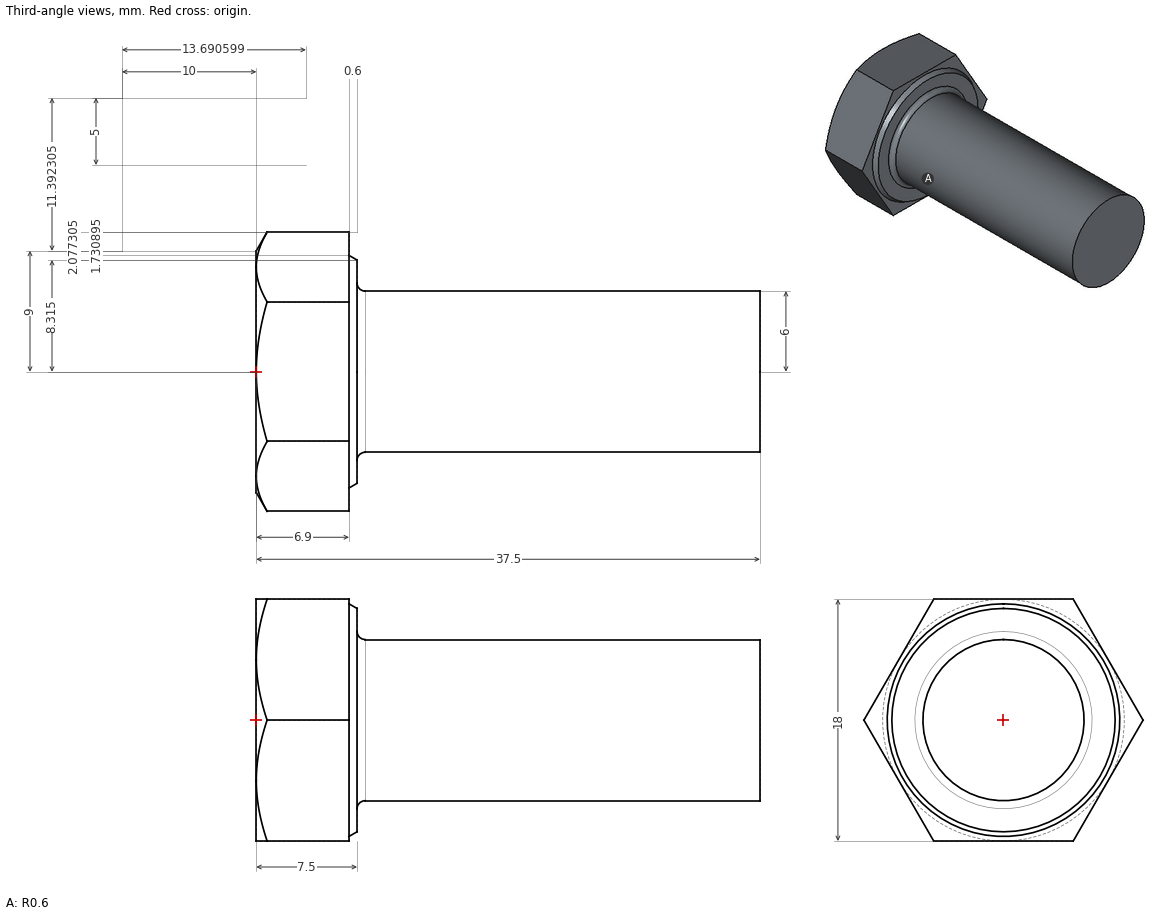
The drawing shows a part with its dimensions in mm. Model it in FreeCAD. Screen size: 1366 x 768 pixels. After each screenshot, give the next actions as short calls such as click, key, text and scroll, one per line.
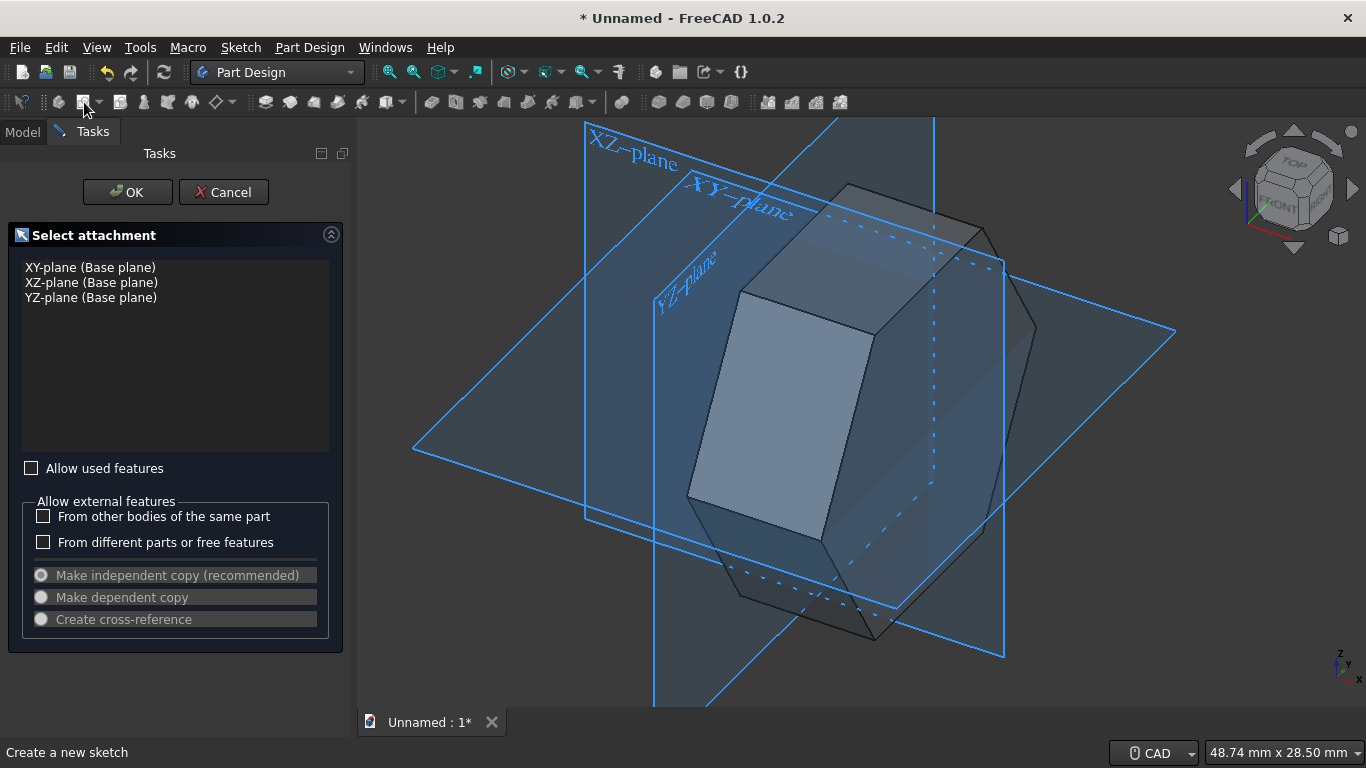
click(82, 268)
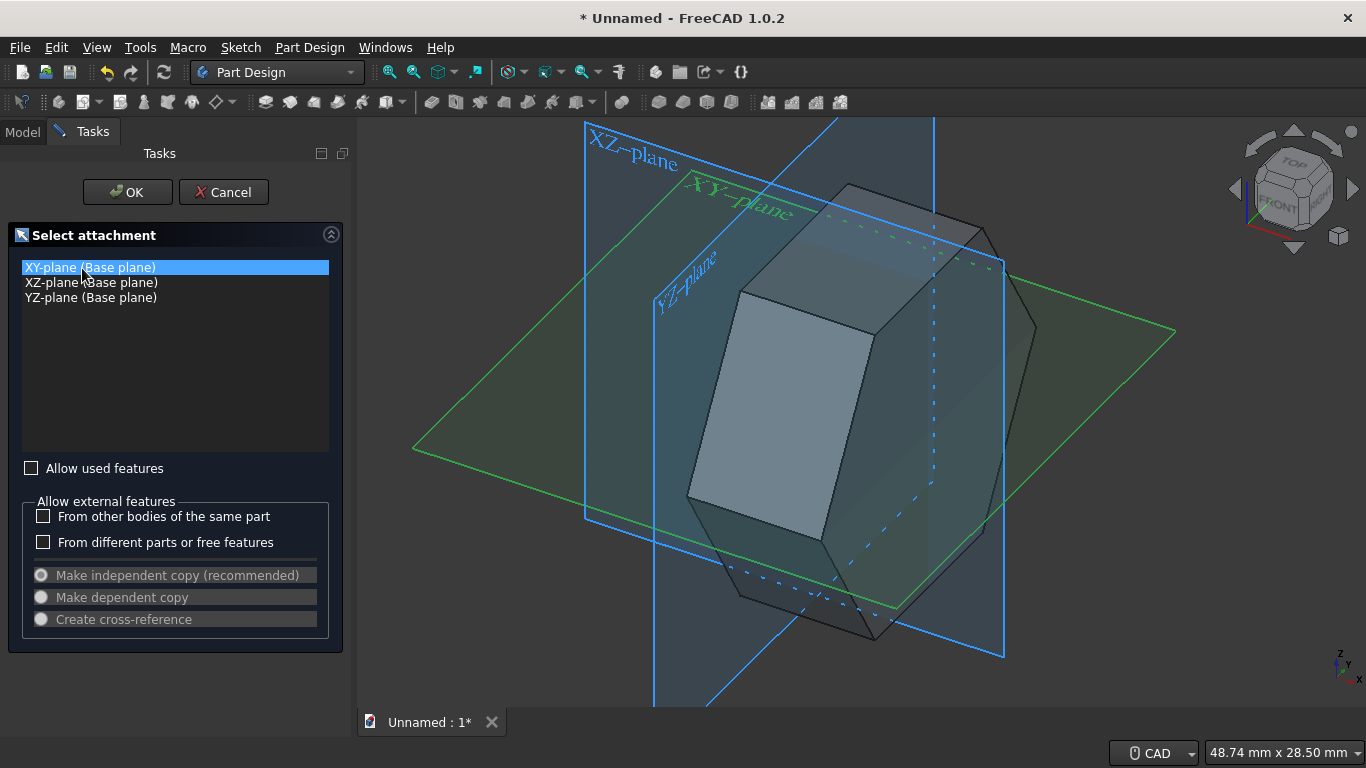
click(128, 192)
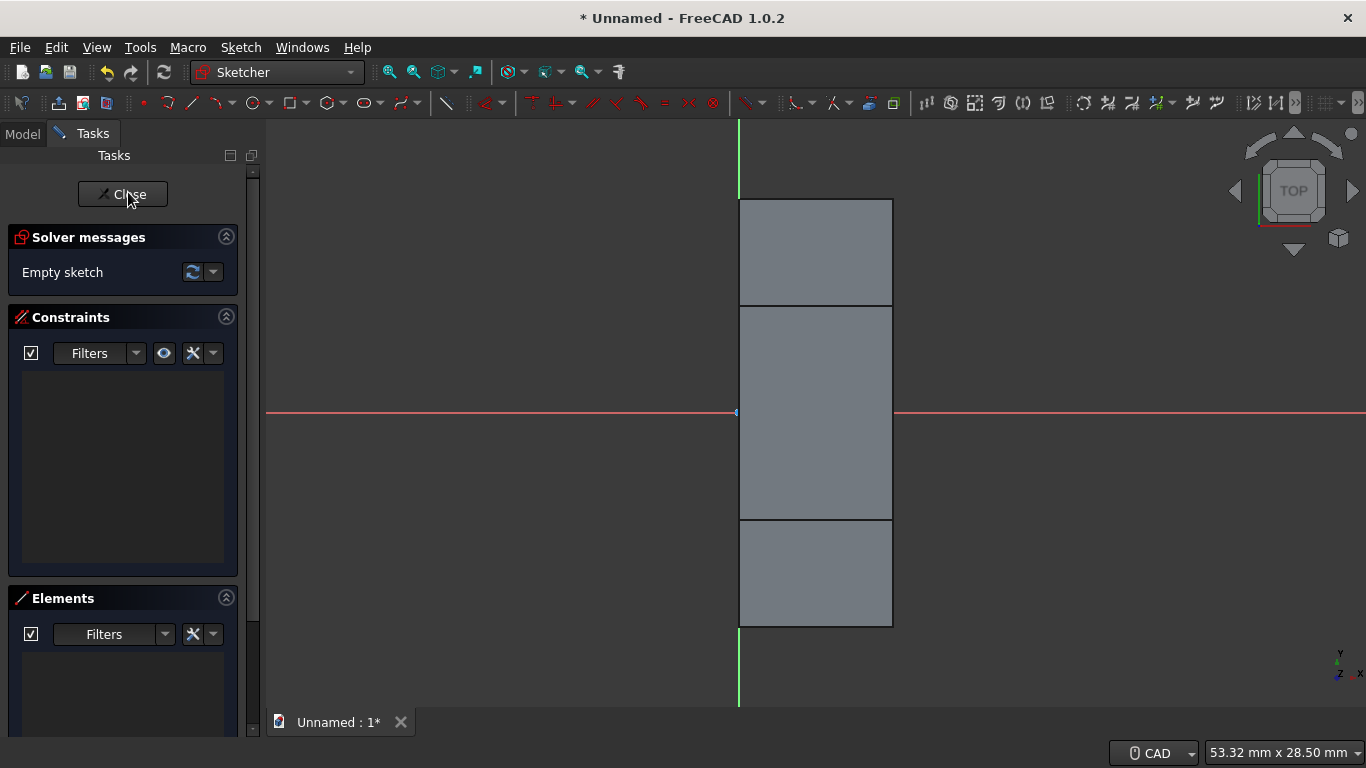
click(108, 104)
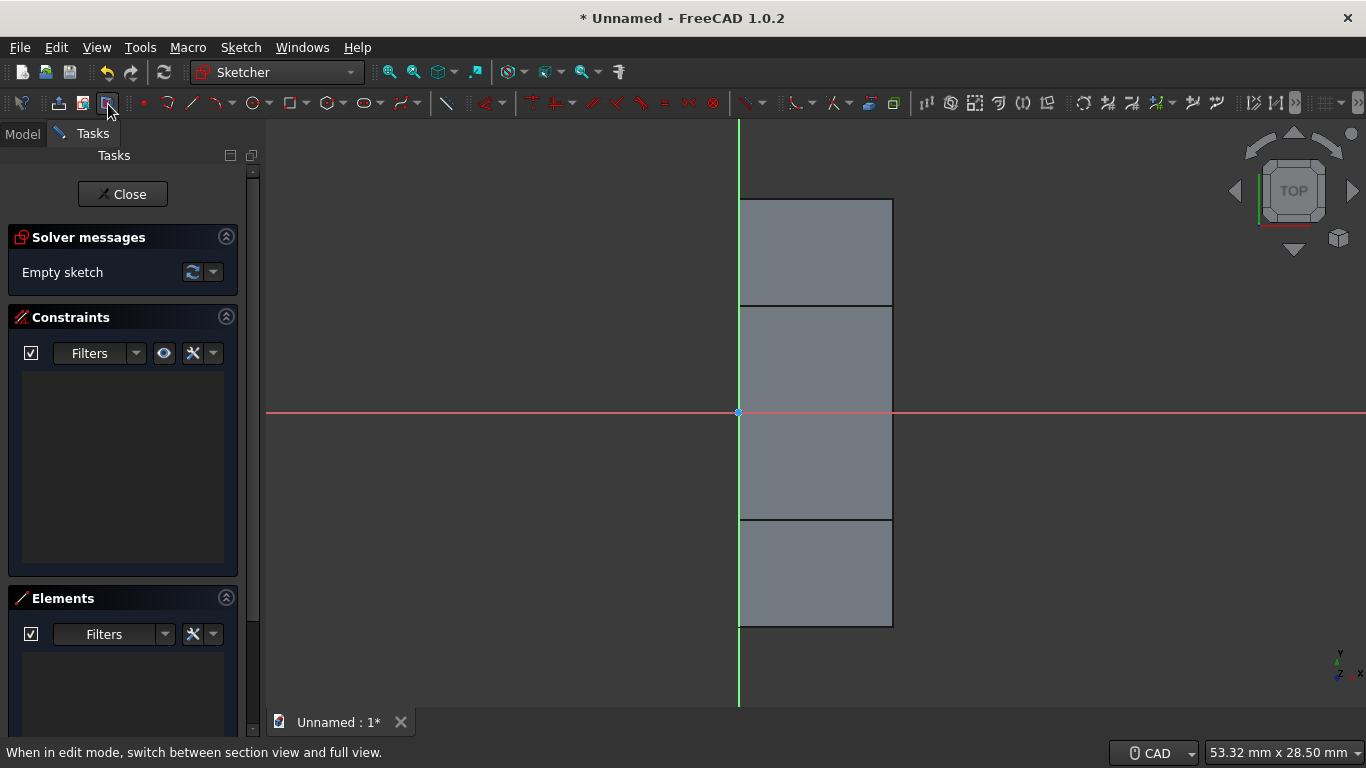
scroll(294, 539, down, 2)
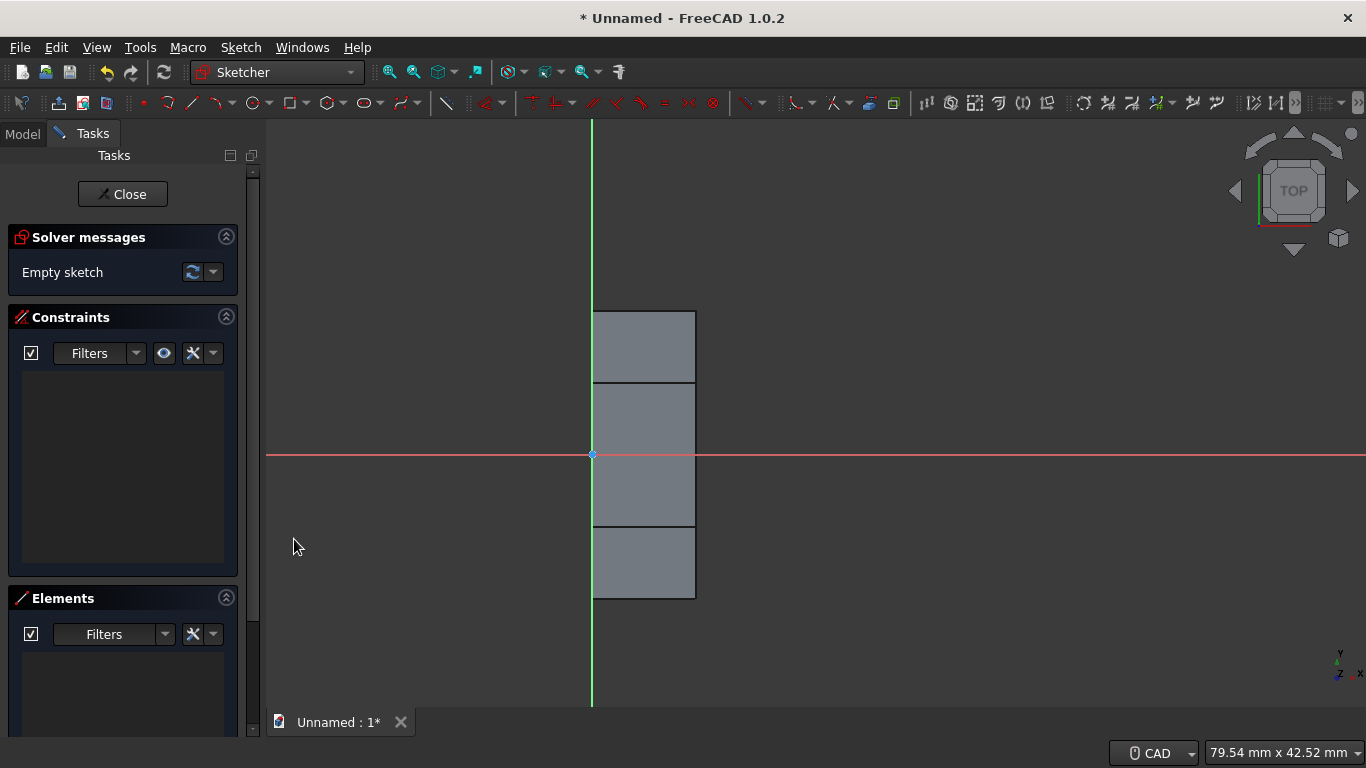
key(g)
key(r)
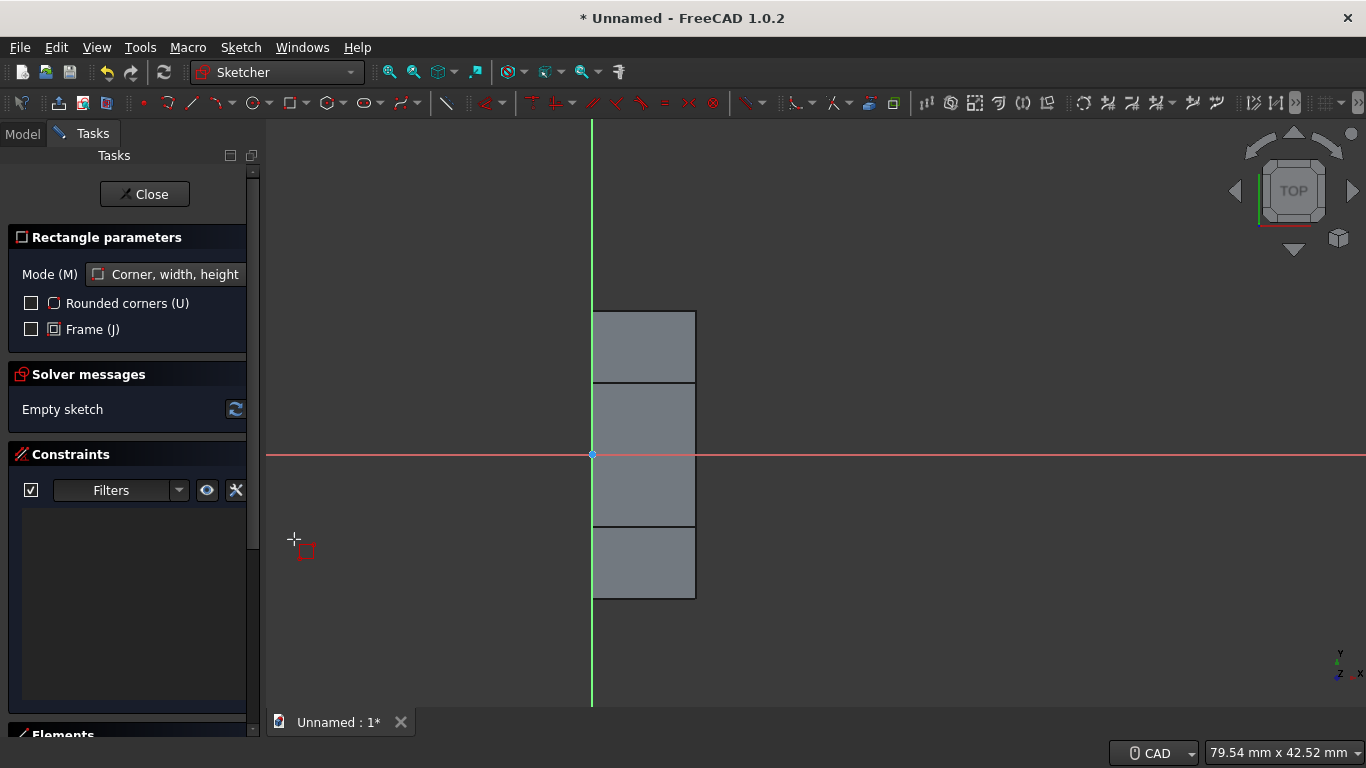
click(592, 455)
move(1111, 372)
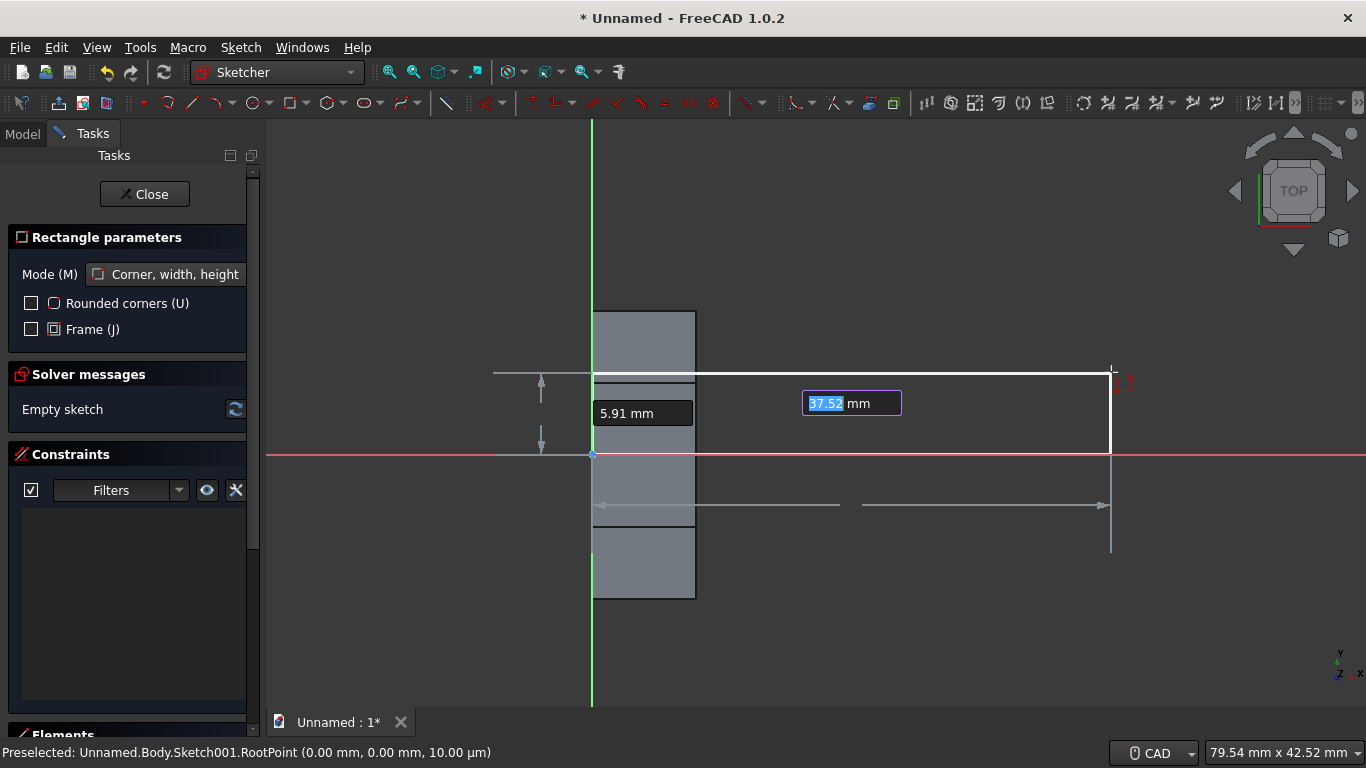
text(37.5)
key(Tab)
text(6)
key(Return)
key(Escape)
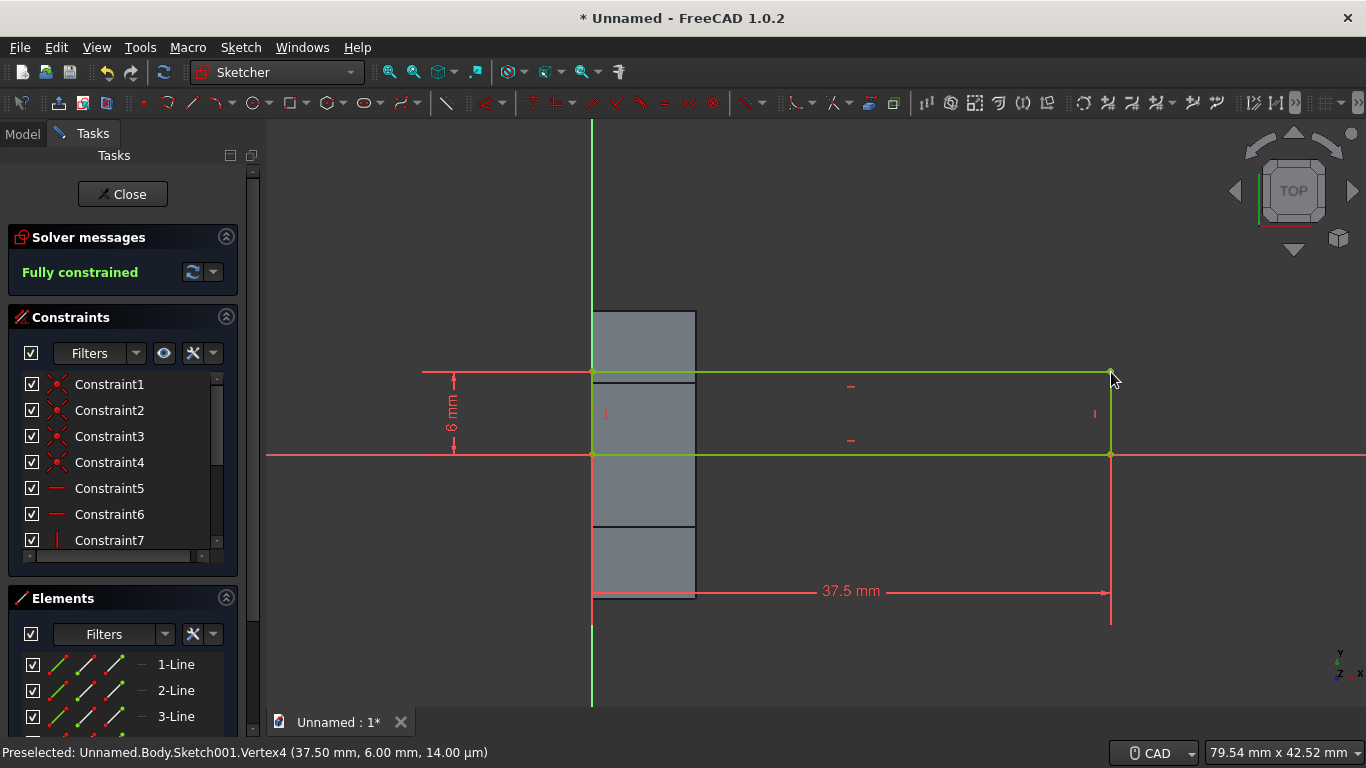
click(123, 194)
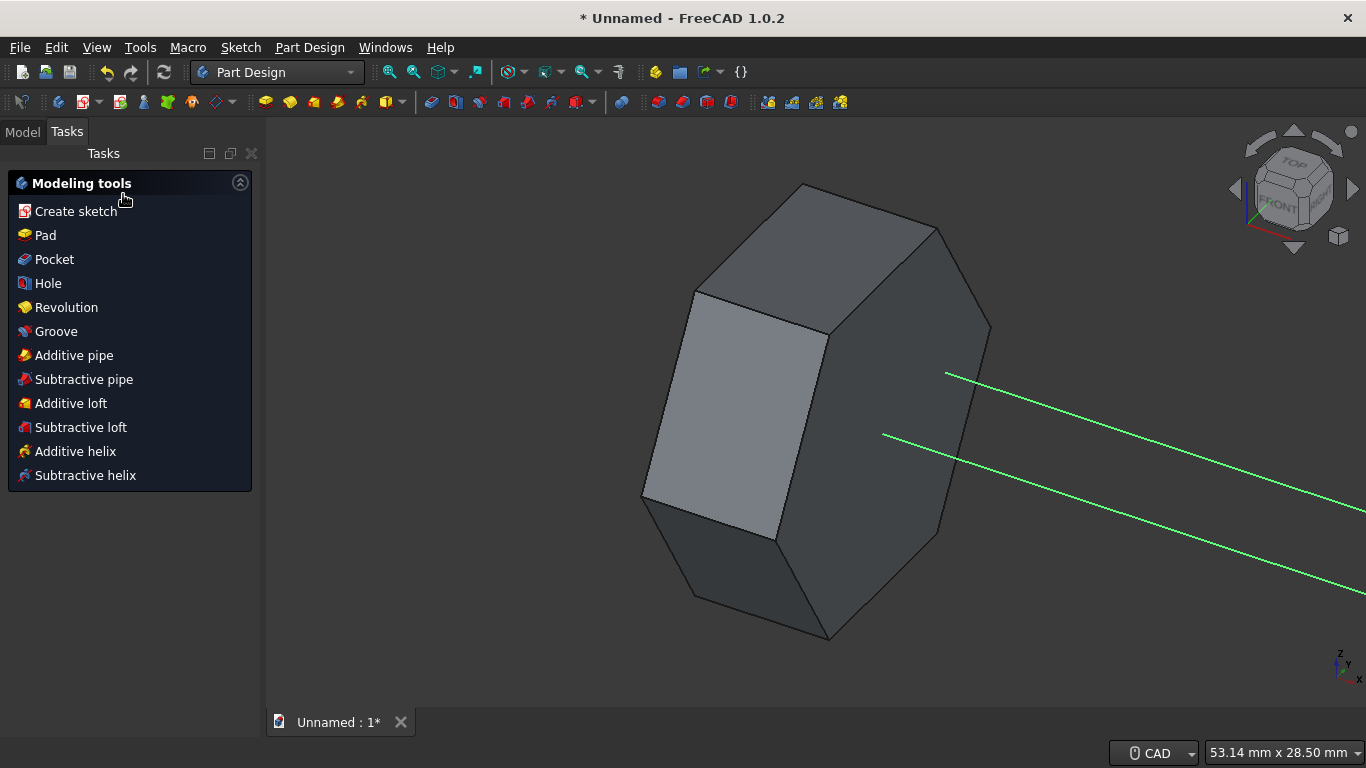
click(290, 102)